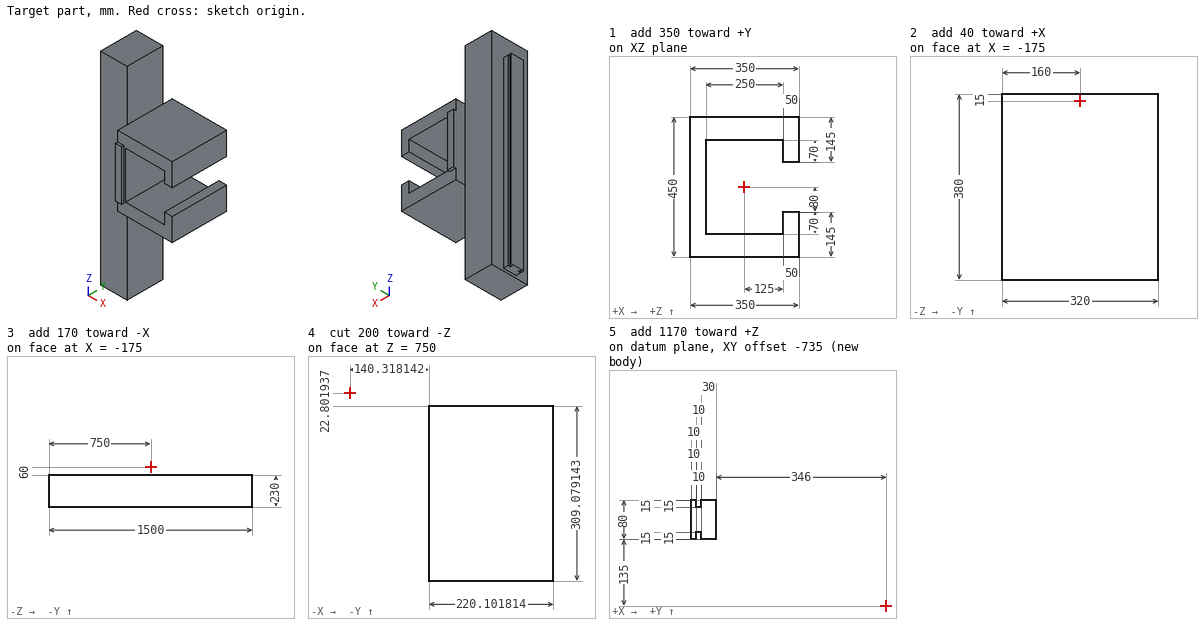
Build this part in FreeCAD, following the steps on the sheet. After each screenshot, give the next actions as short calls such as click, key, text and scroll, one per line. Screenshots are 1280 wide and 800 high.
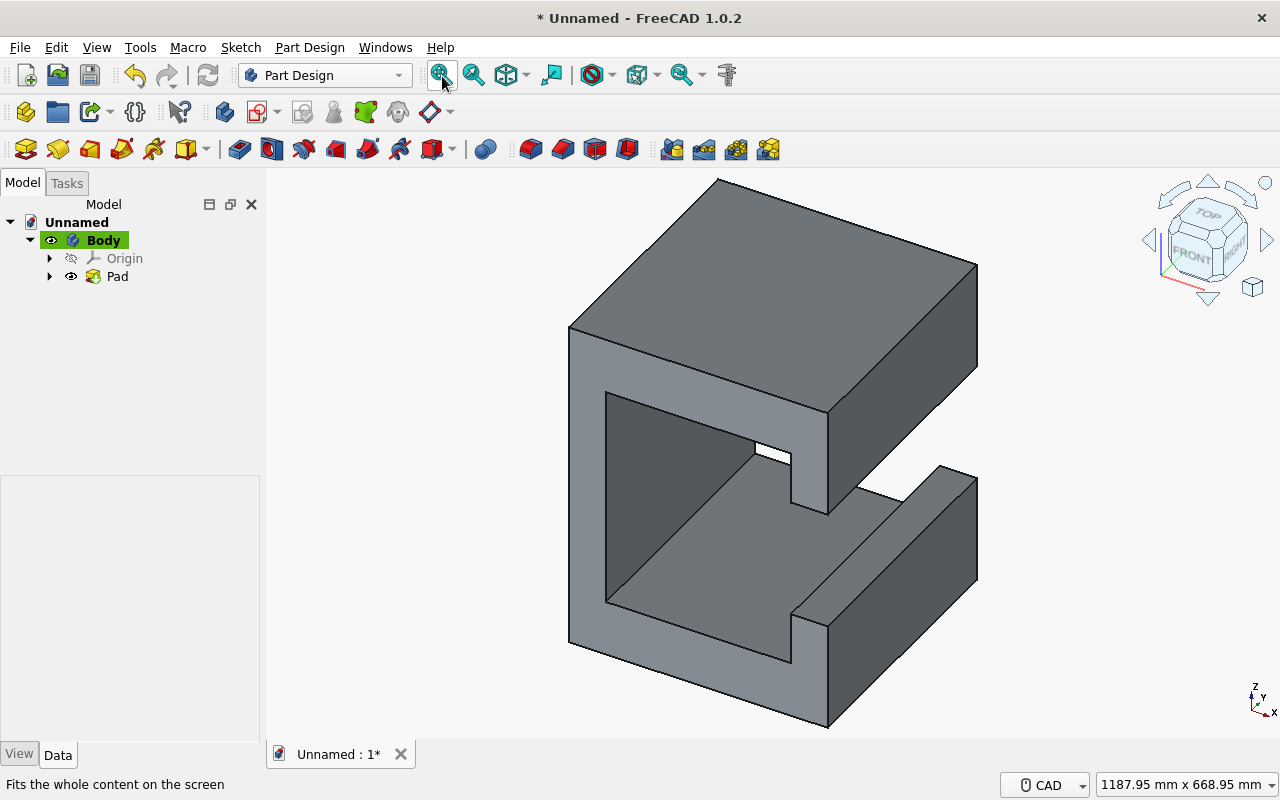
key(6)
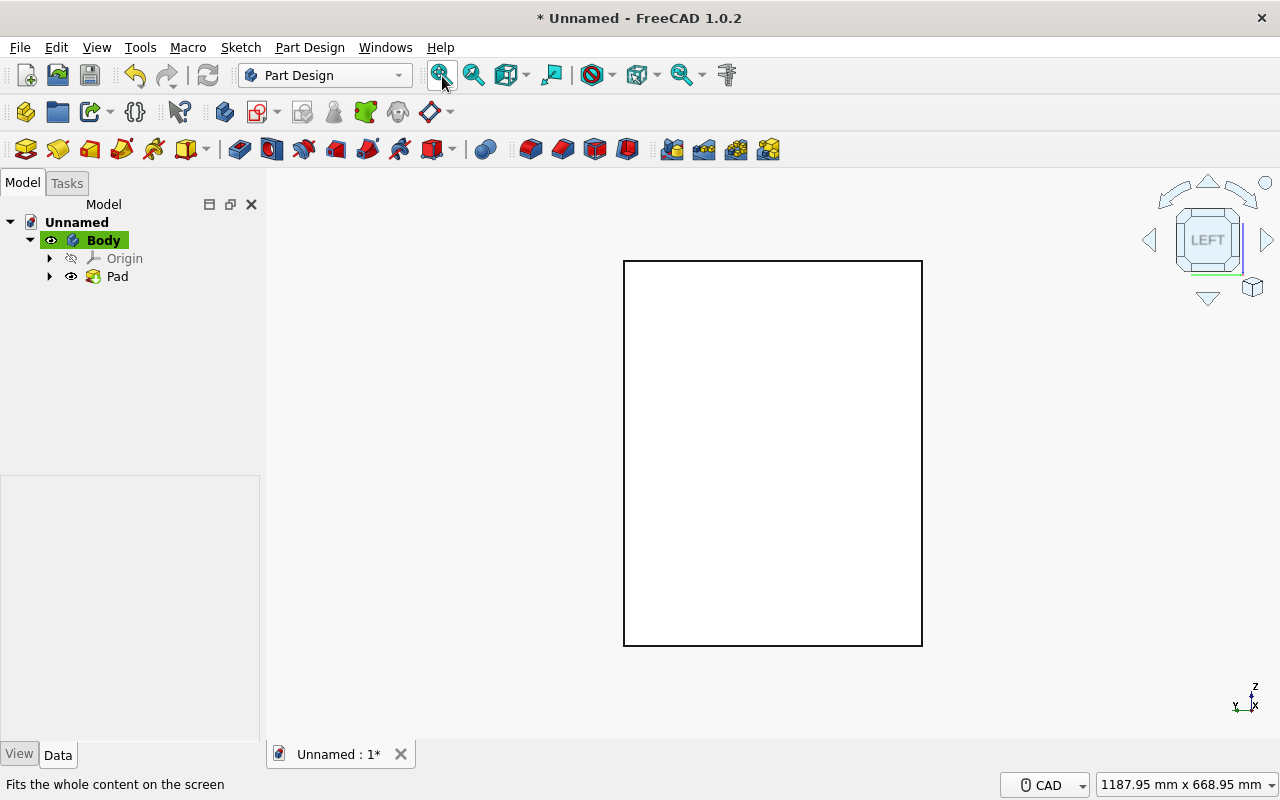
click(773, 453)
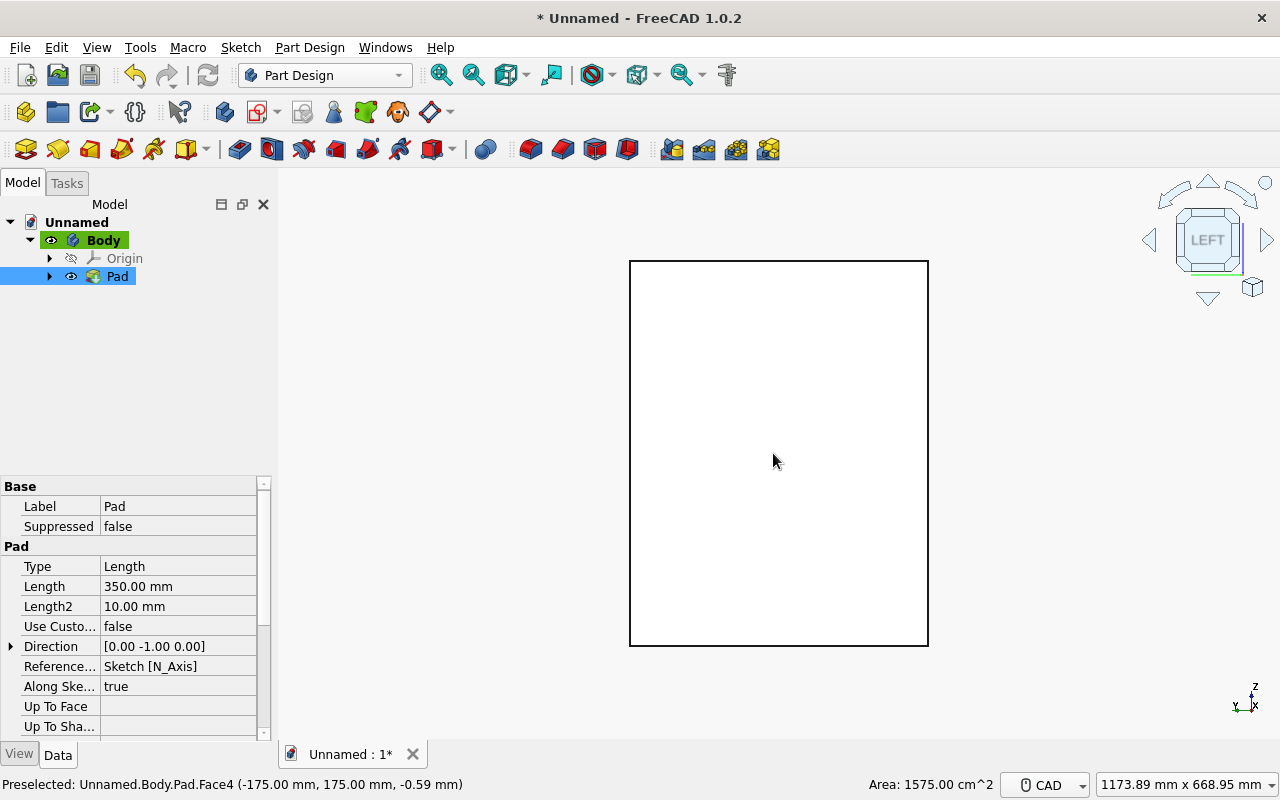
click(258, 112)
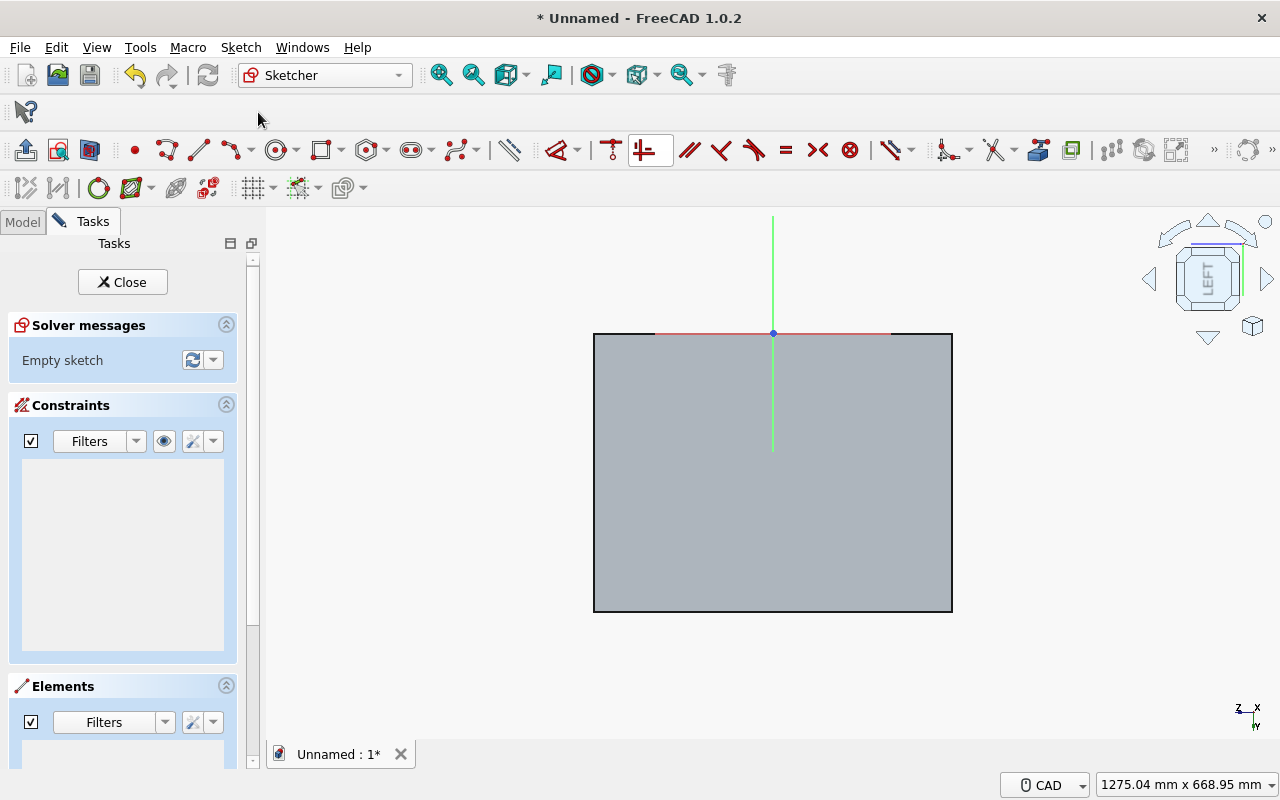
click(322, 150)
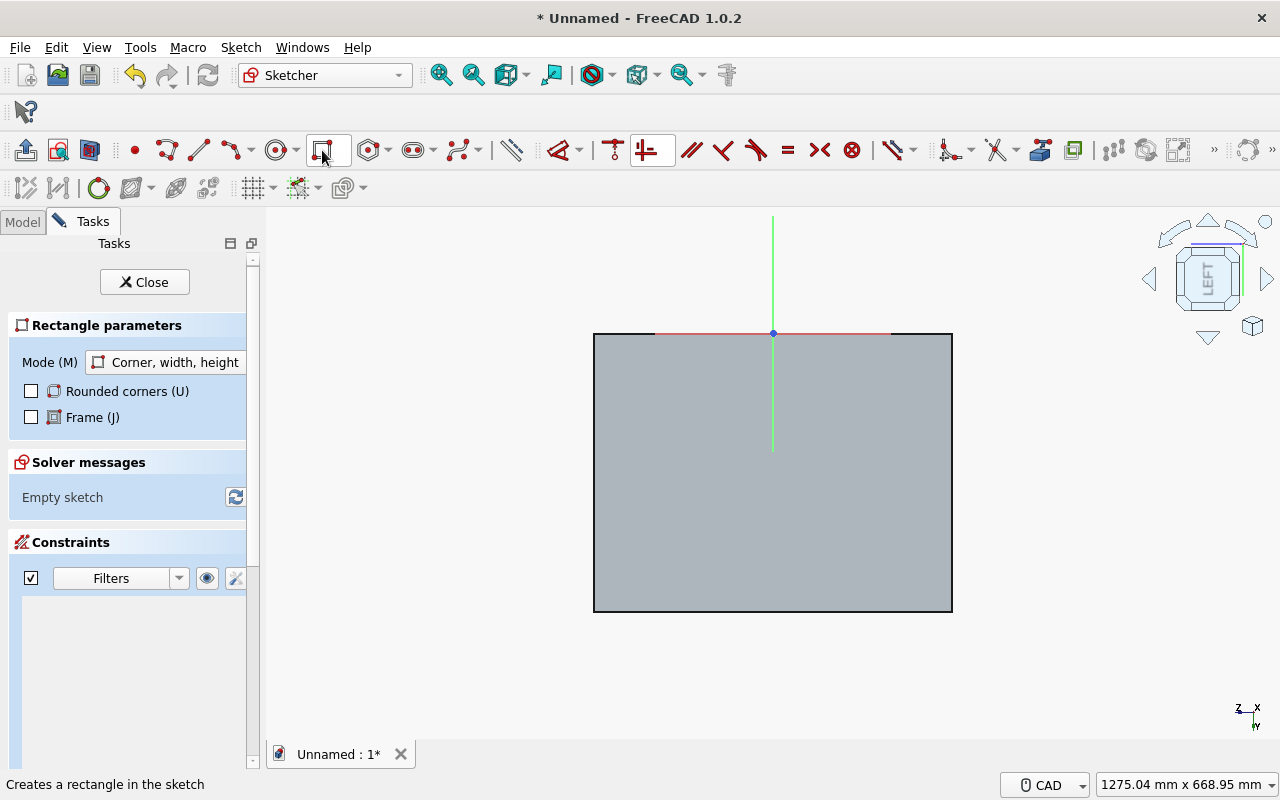
scroll(646, 322, up, 2)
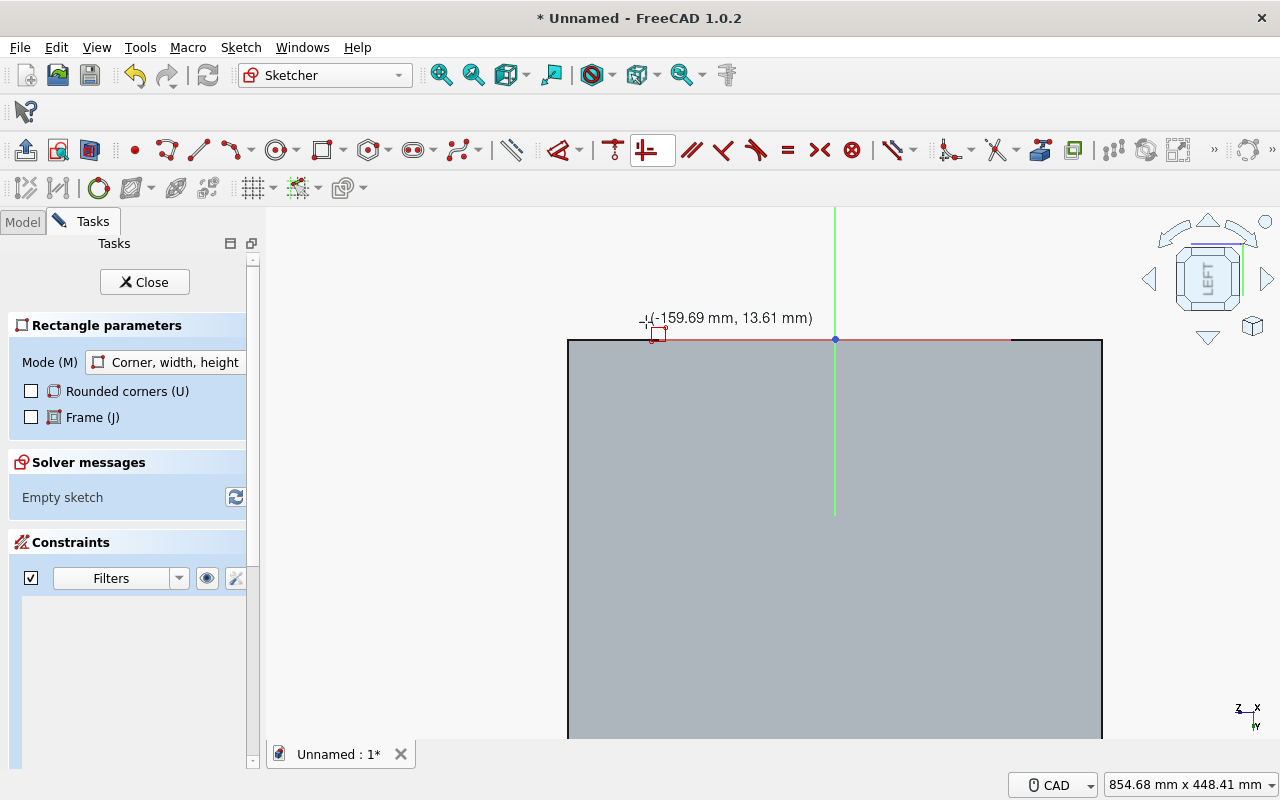
click(645, 322)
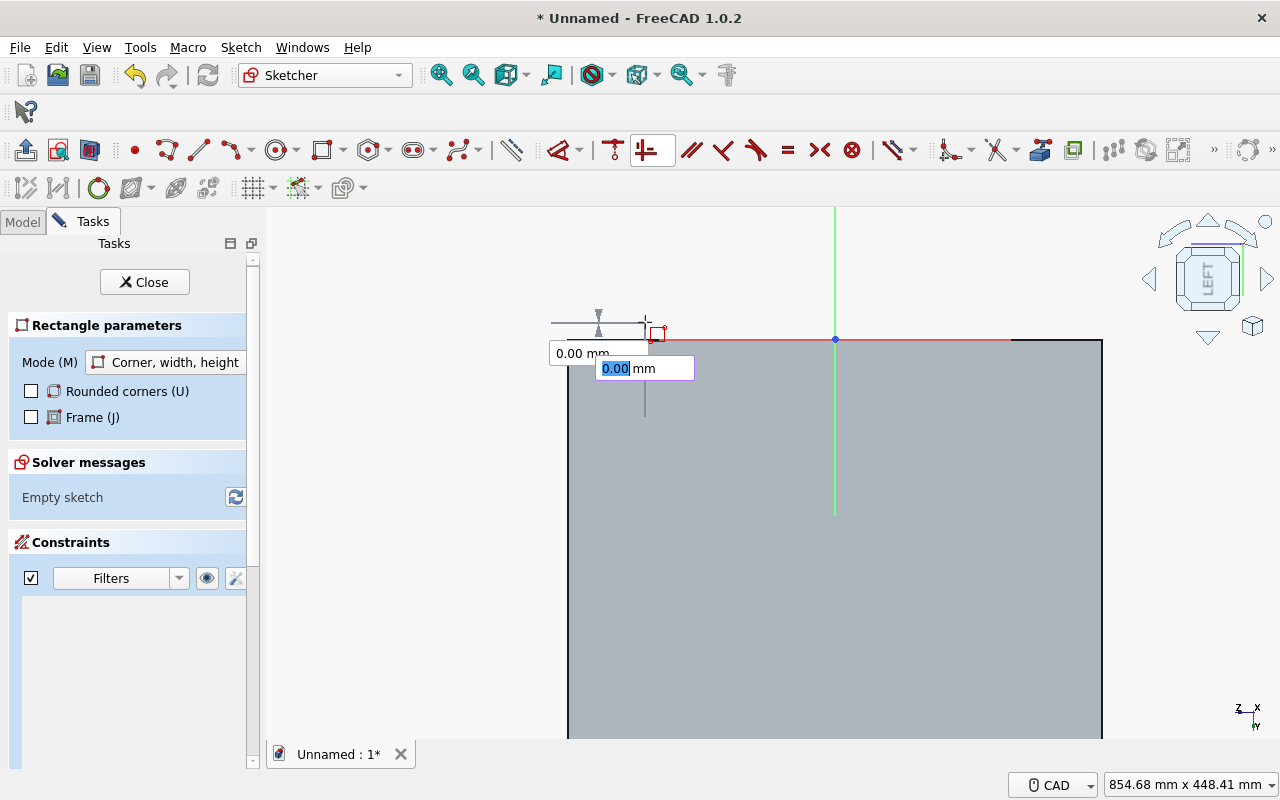
scroll(294, 235, down, 1)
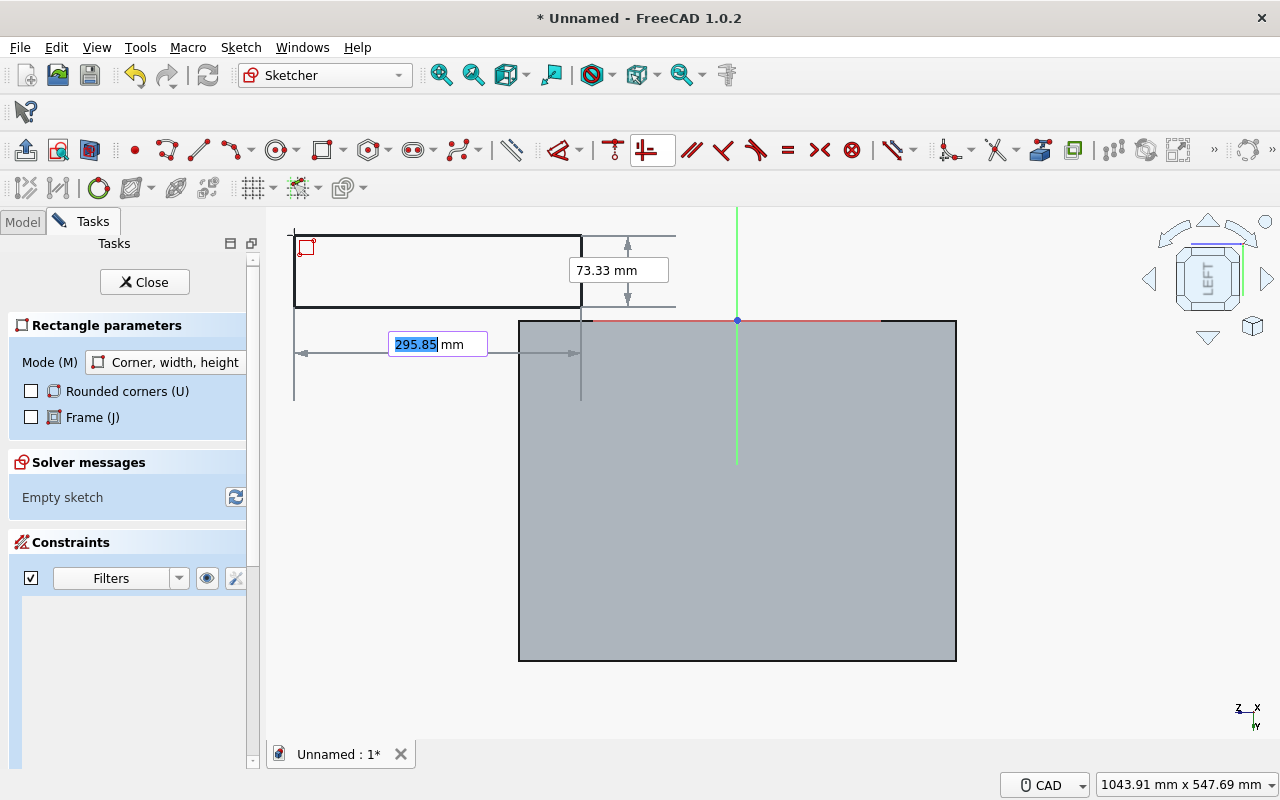
click(893, 675)
key(Escape)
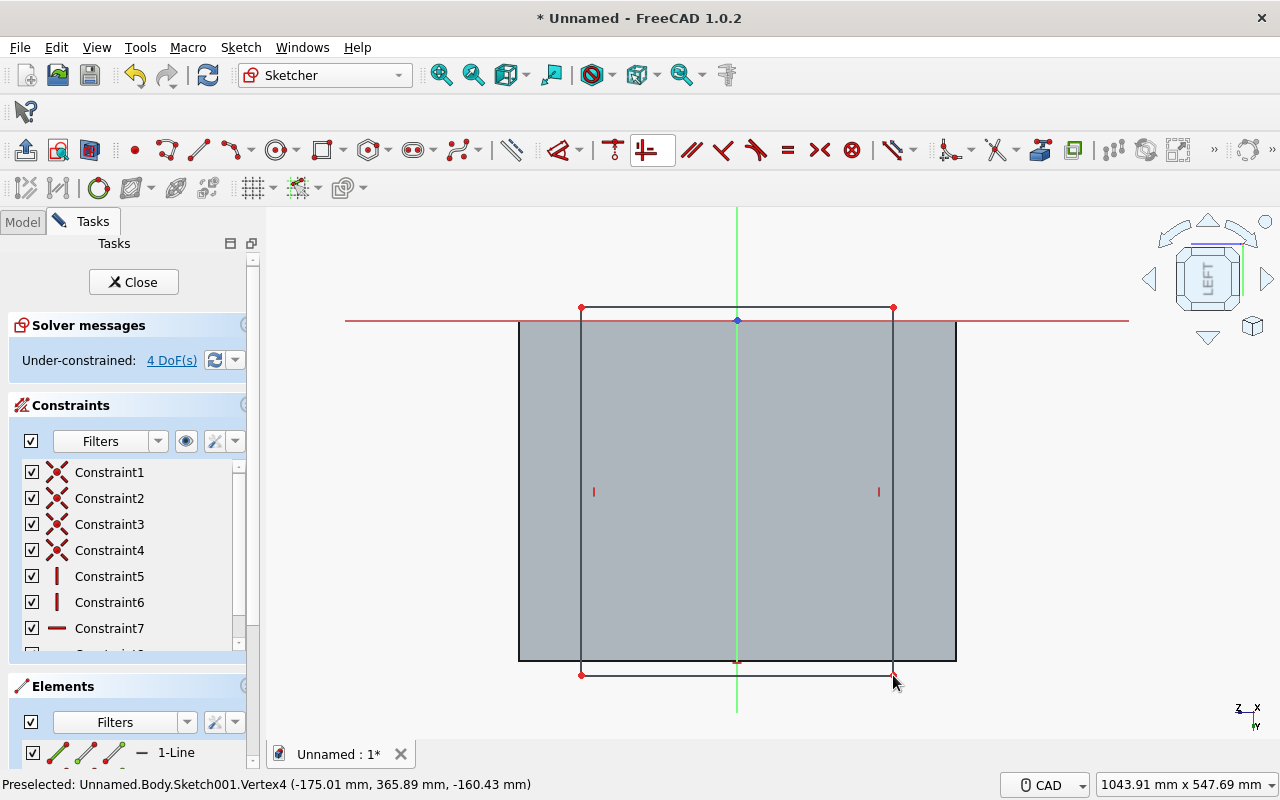
click(558, 150)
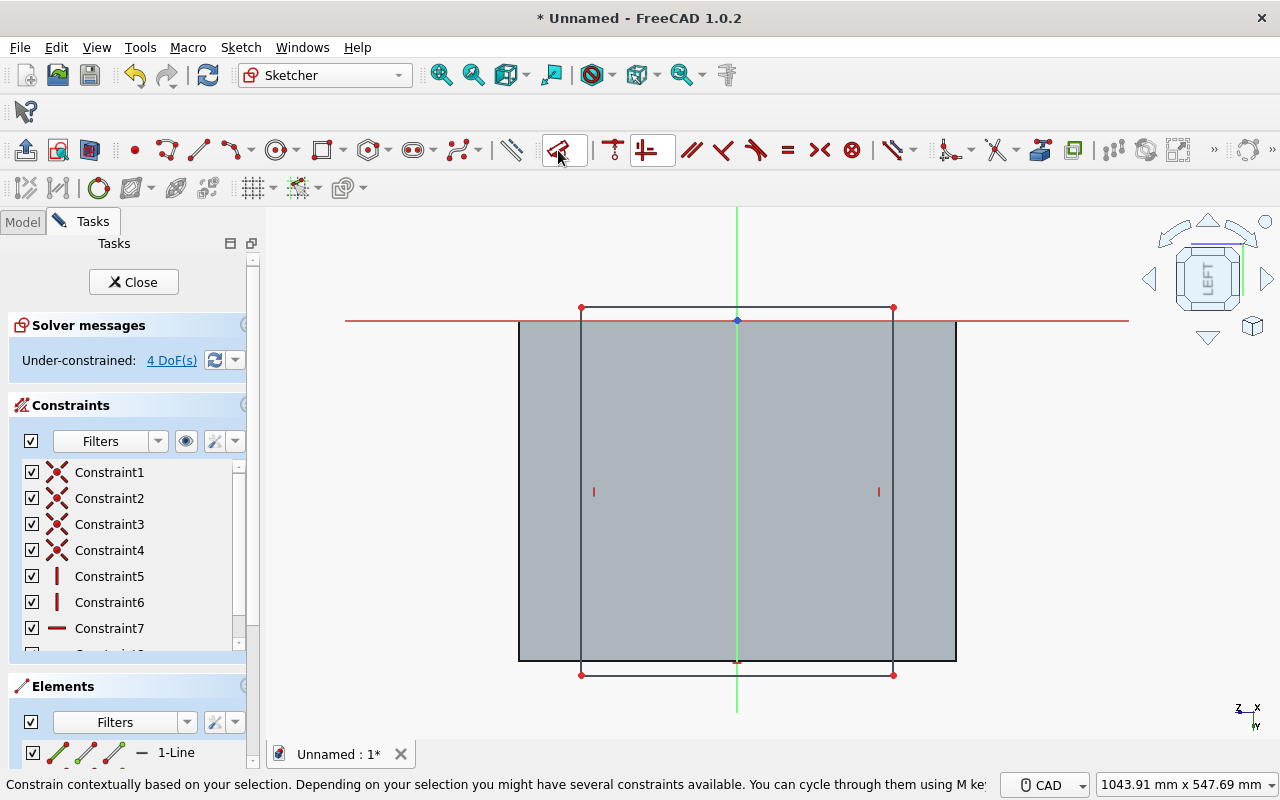
click(581, 418)
click(547, 492)